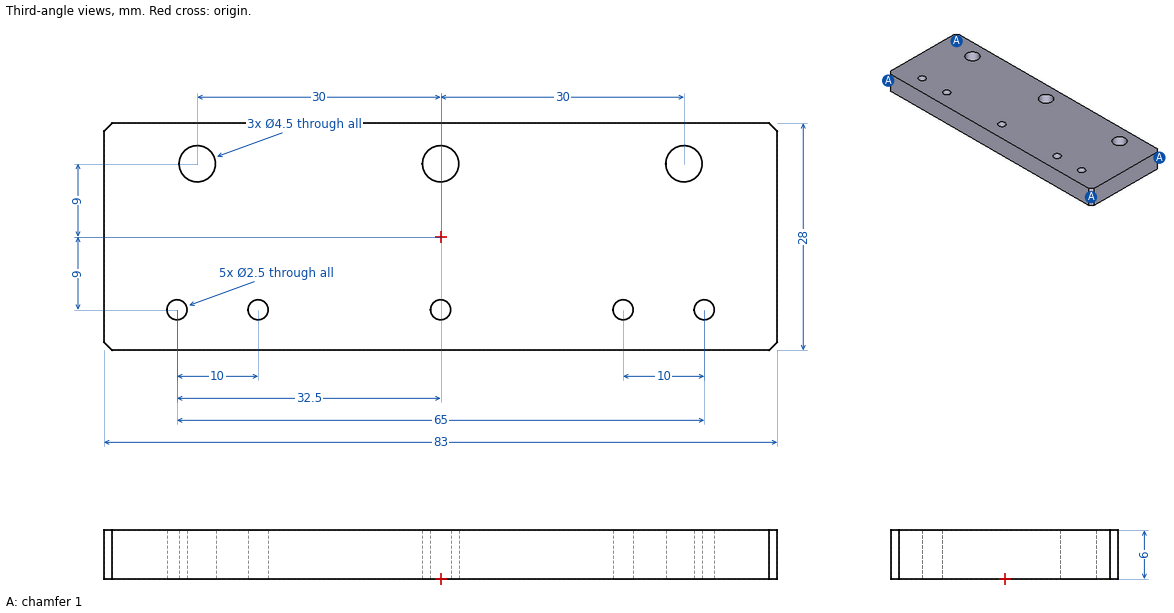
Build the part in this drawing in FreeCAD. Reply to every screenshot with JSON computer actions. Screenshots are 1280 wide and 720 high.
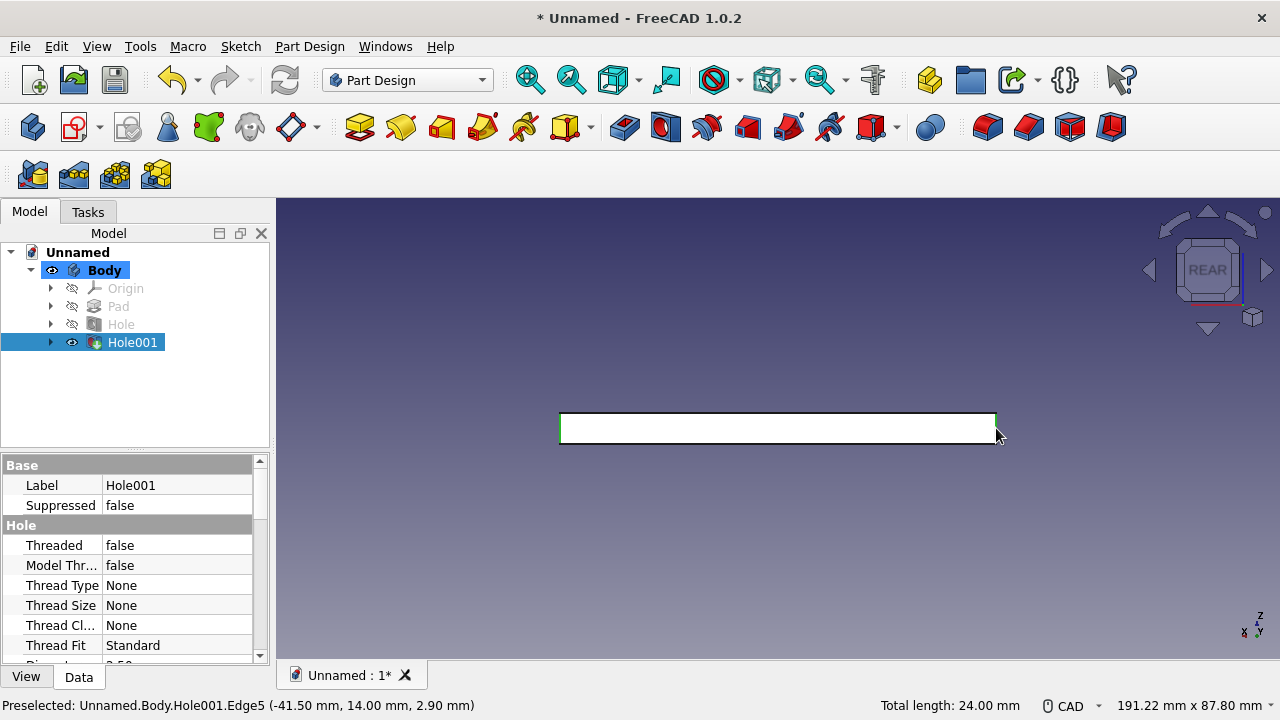
{"action": "left_click", "coordinate": [1029, 128]}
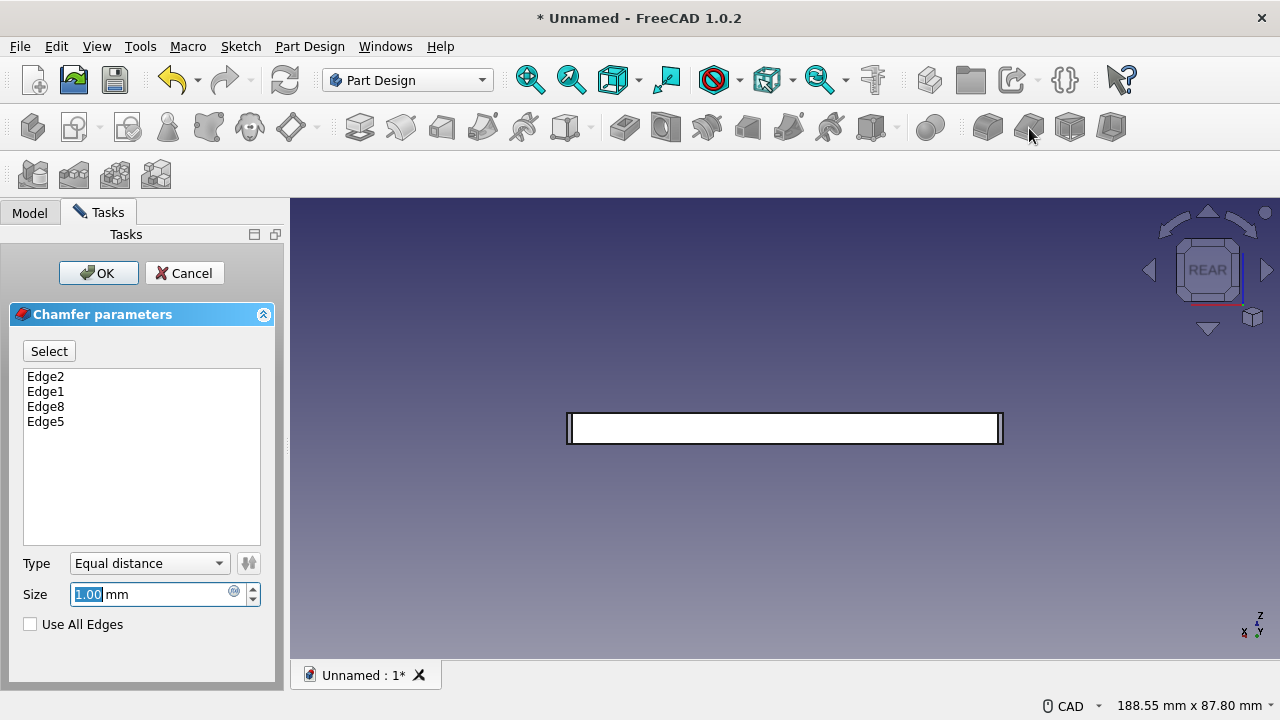
{"action": "type", "text": "1"}
{"action": "key", "text": "Tab"}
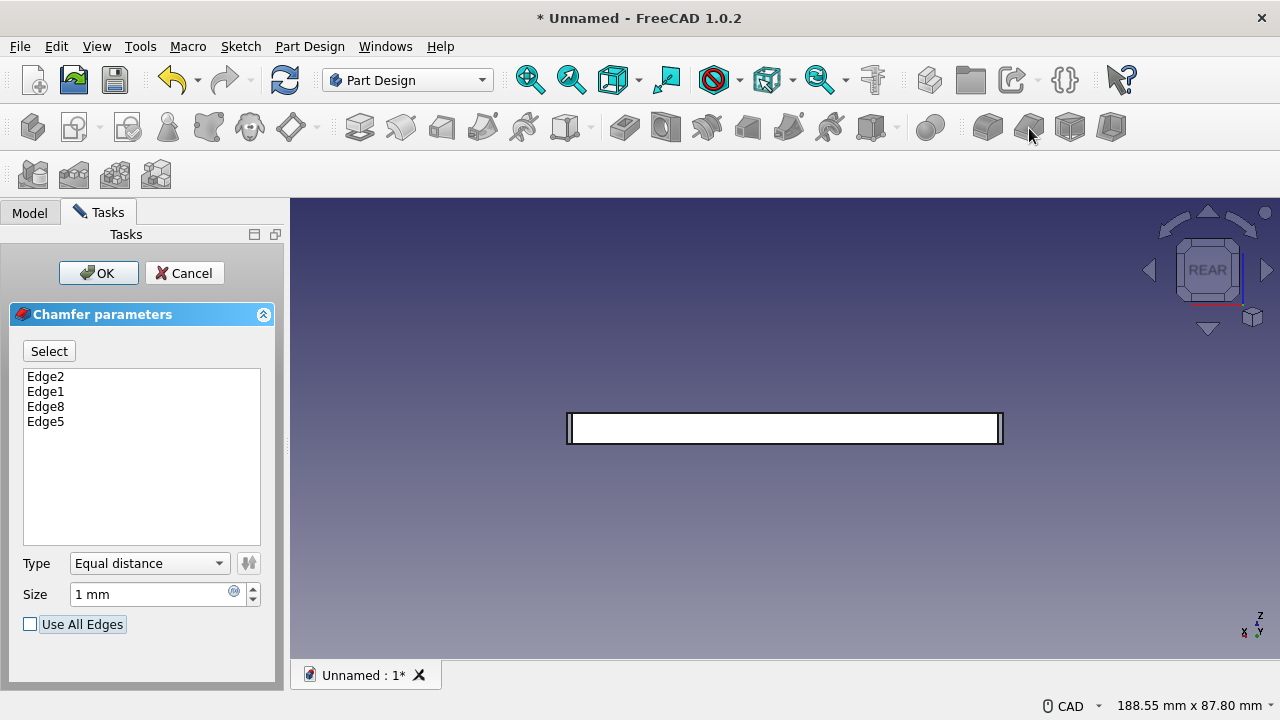
{"action": "left_click", "coordinate": [99, 273]}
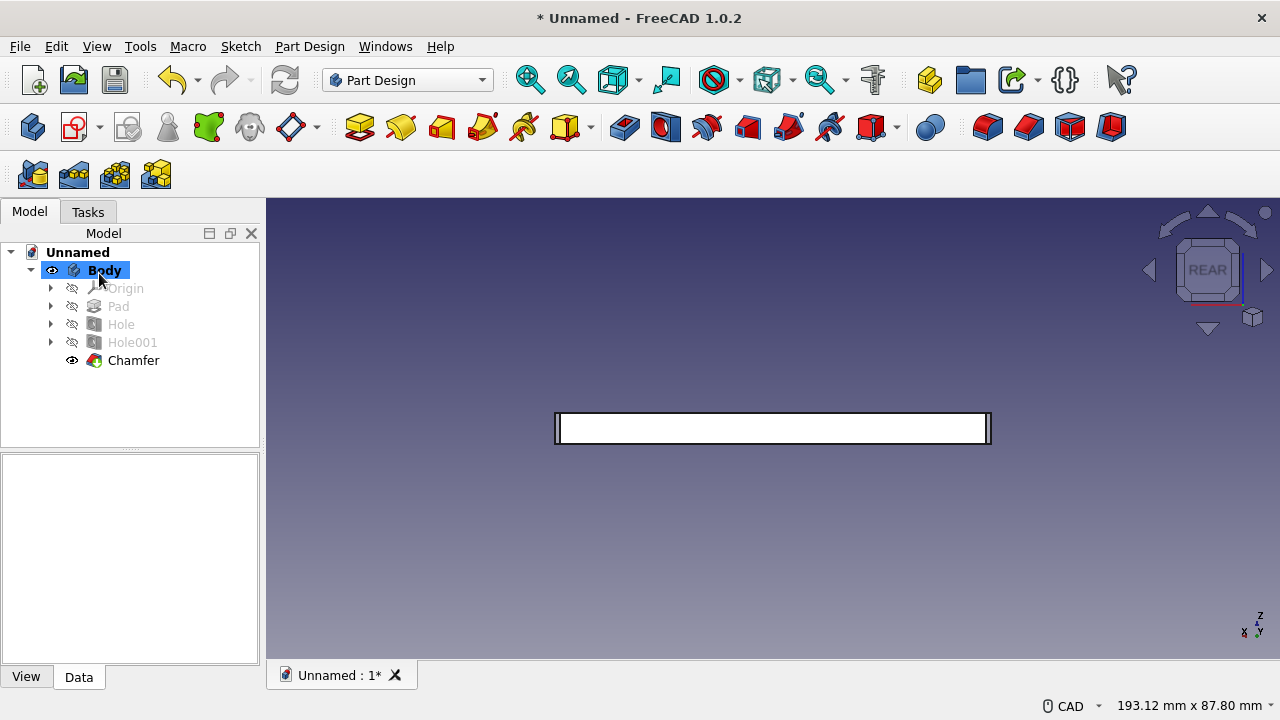
{"action": "key", "text": "0"}